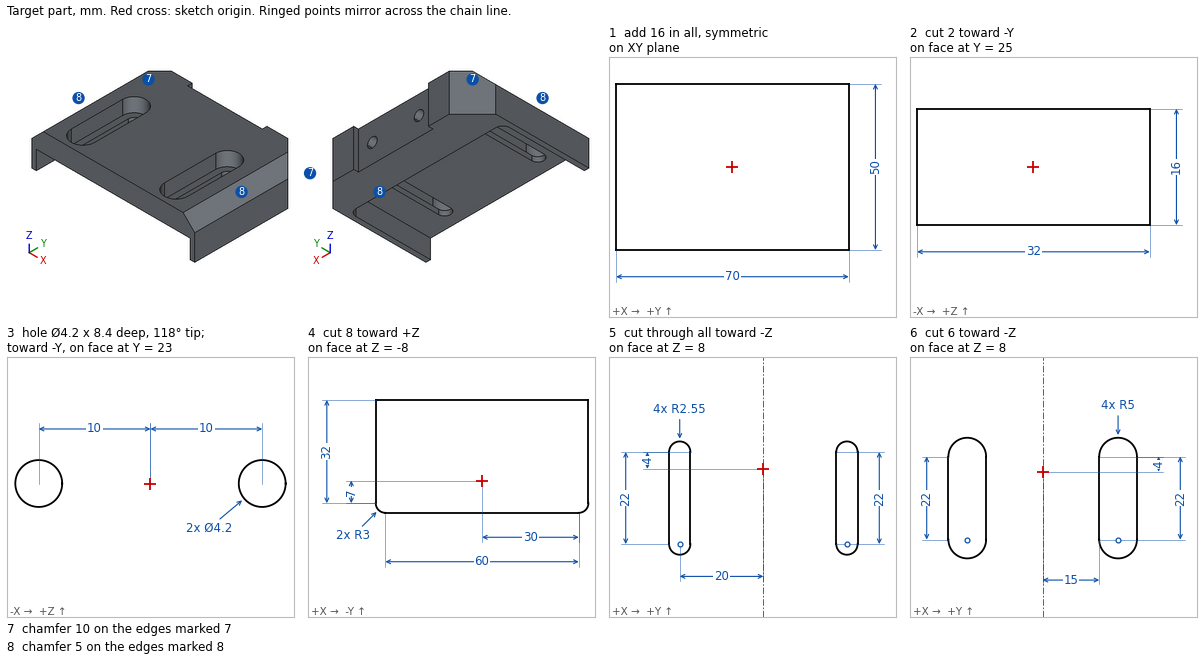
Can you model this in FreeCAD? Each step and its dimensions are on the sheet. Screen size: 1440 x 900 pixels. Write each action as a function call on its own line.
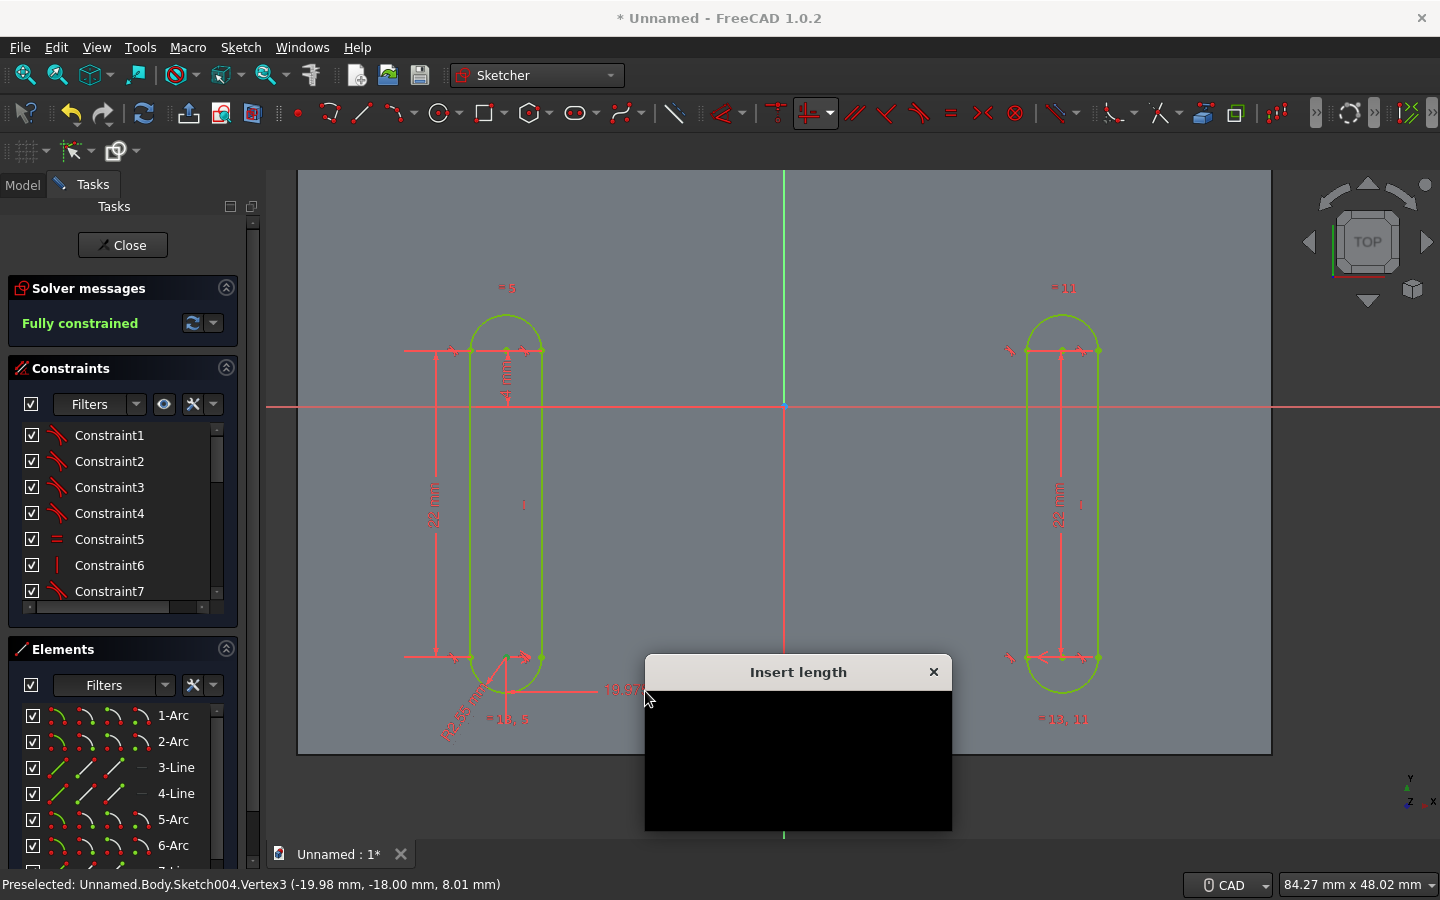
text(20)
key(Return)
key(Escape)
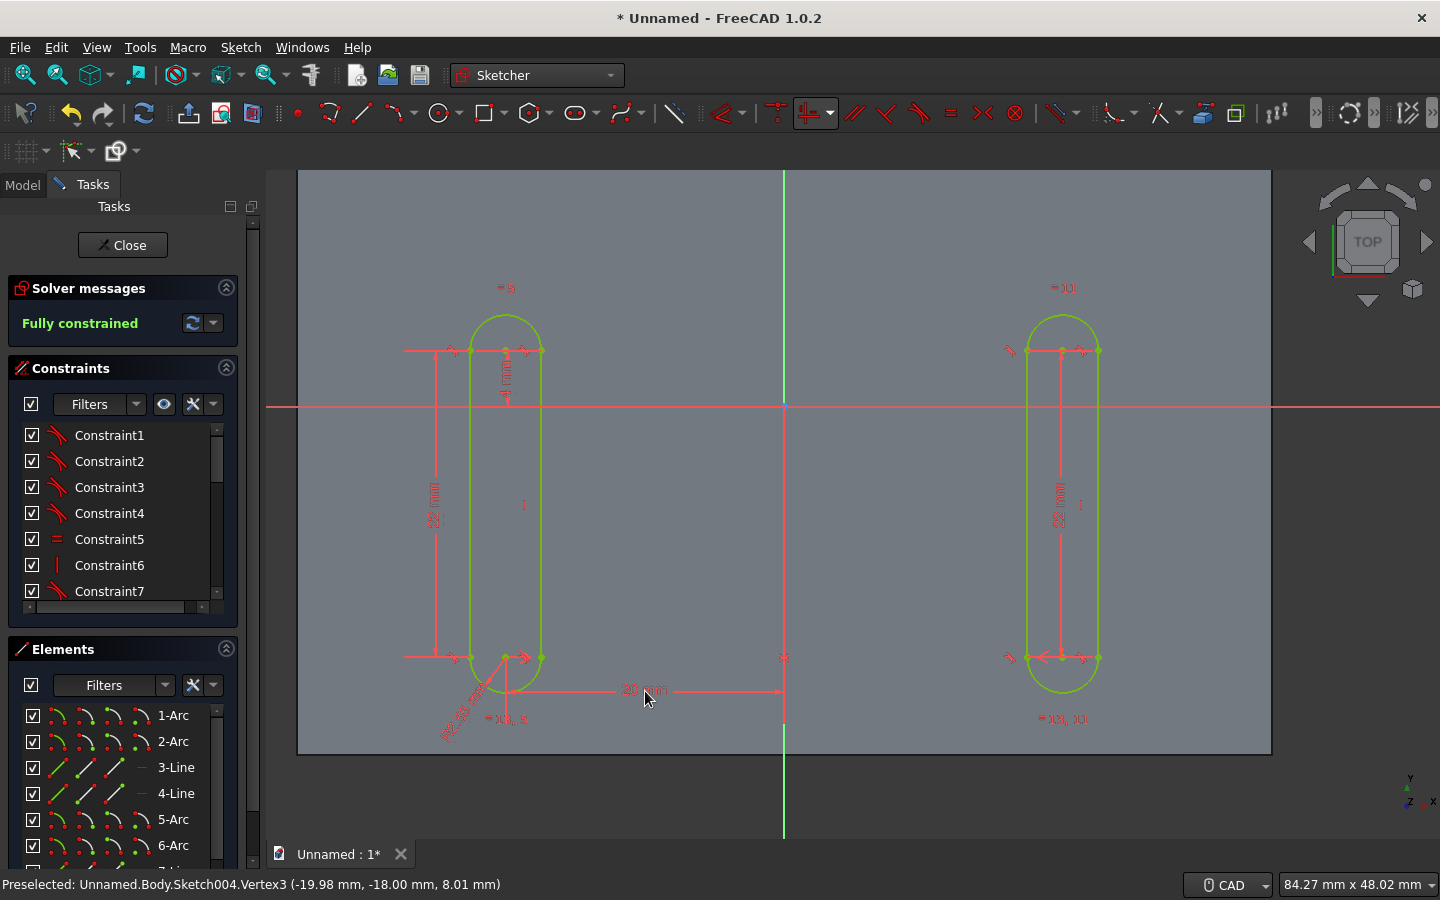
click(123, 245)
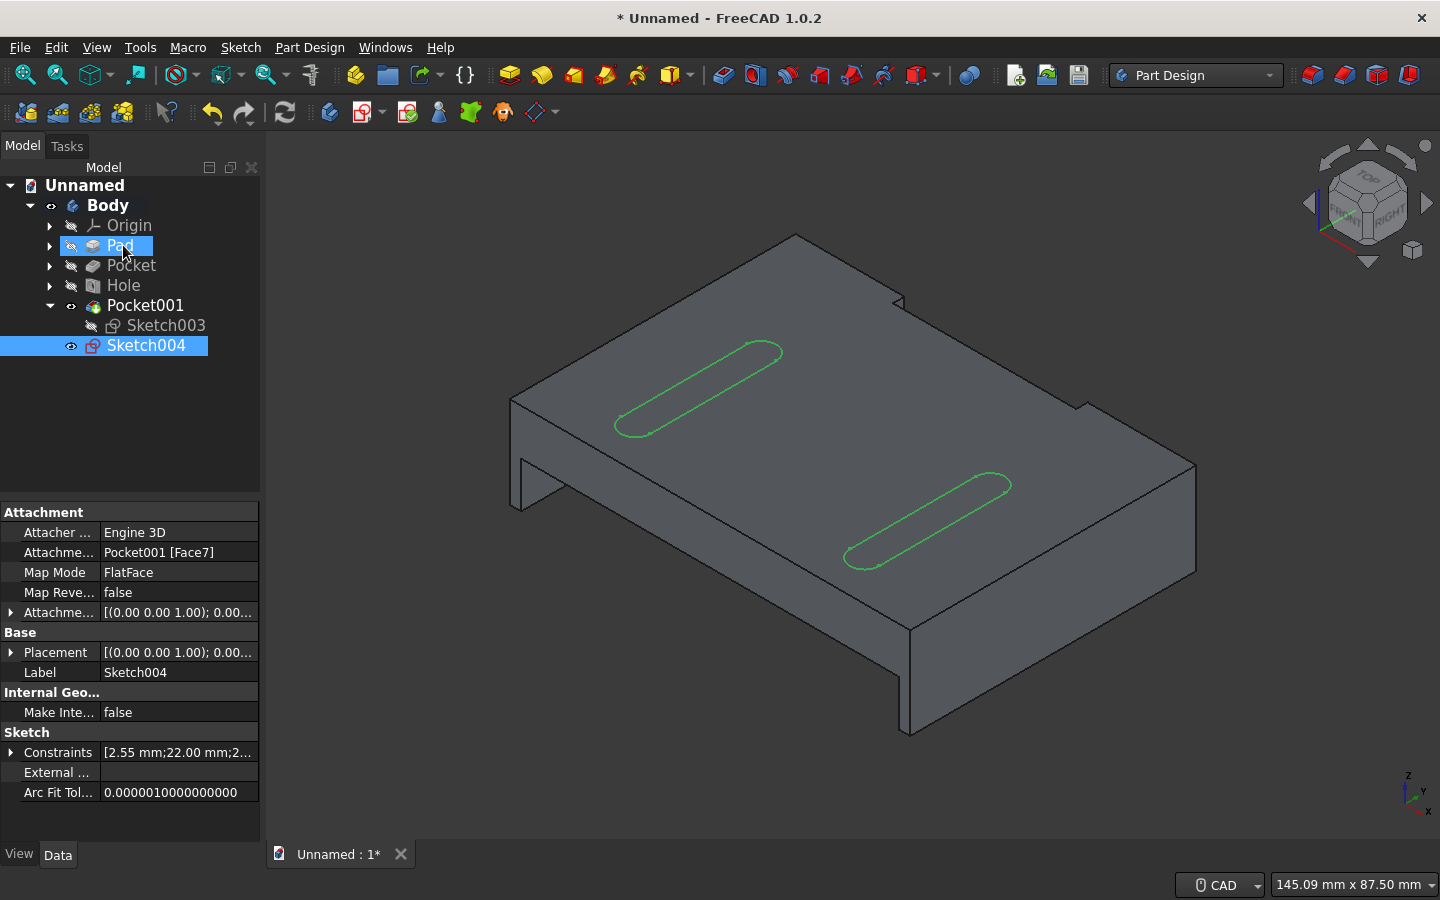
click(724, 76)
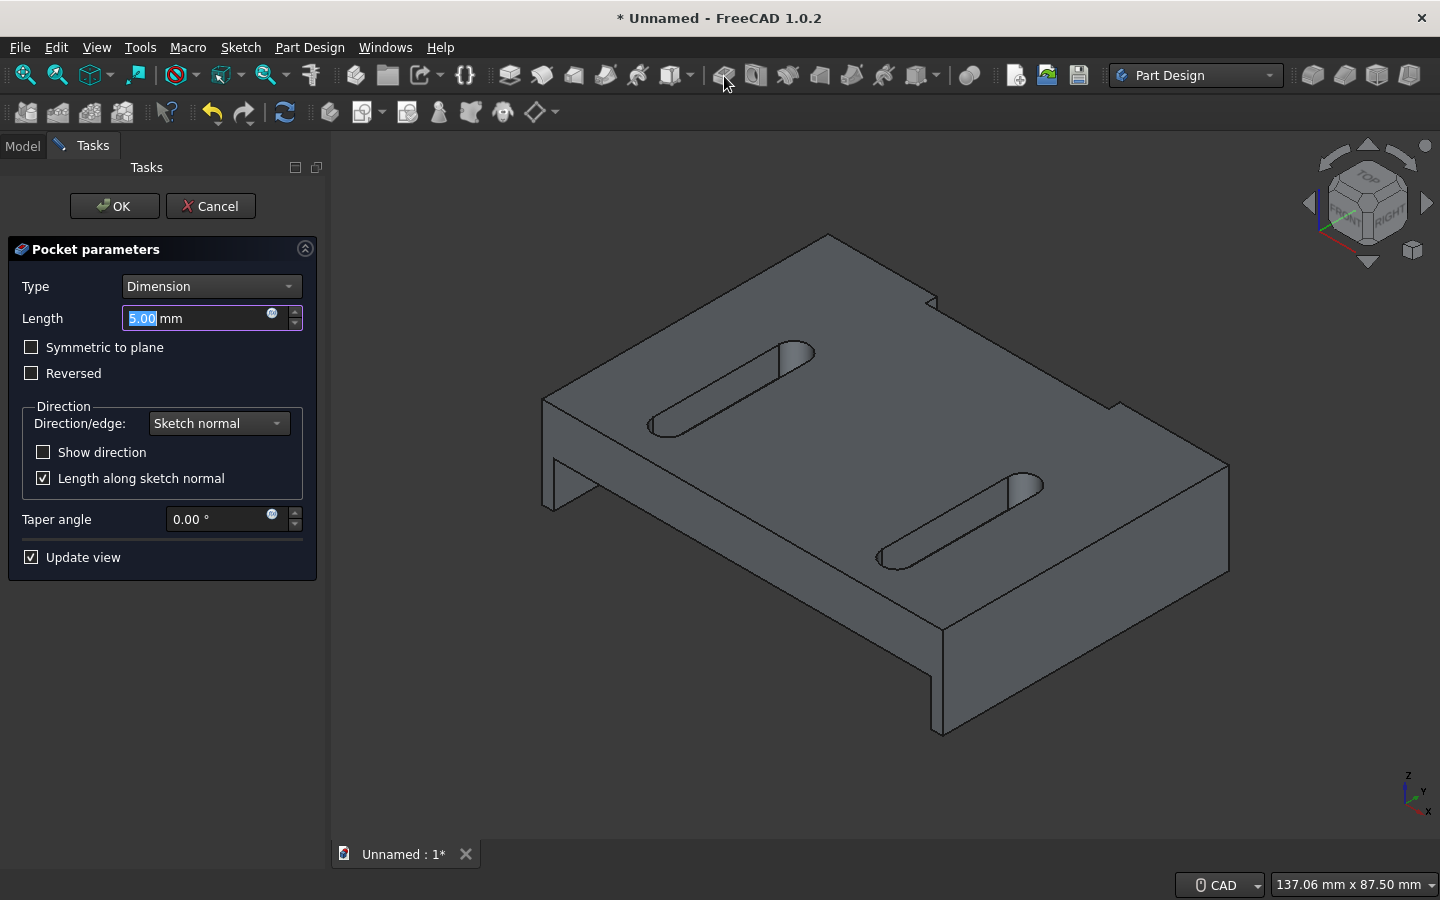
click(212, 286)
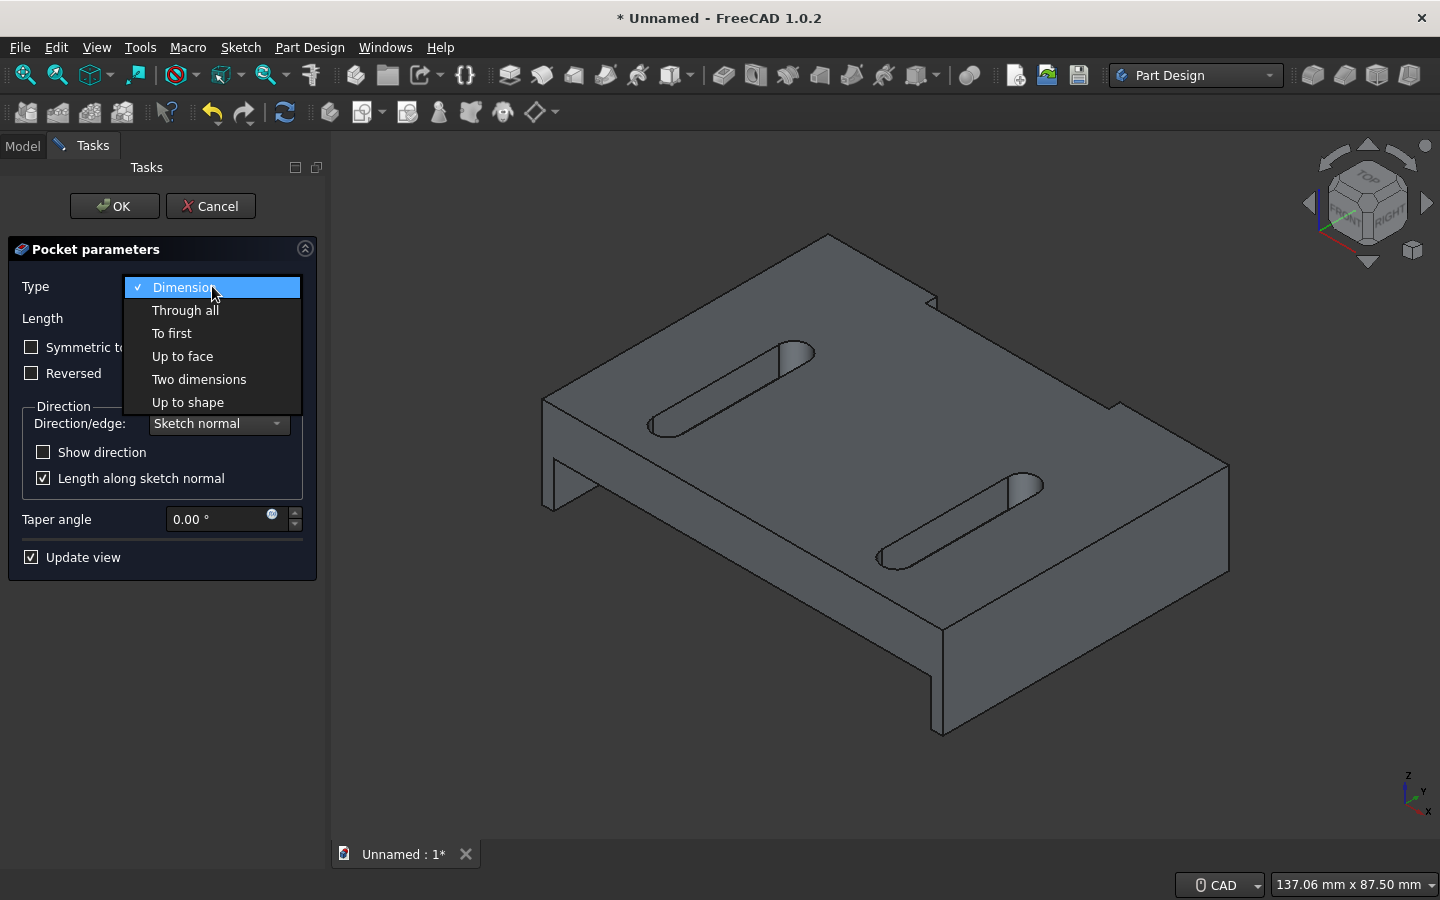
click(212, 310)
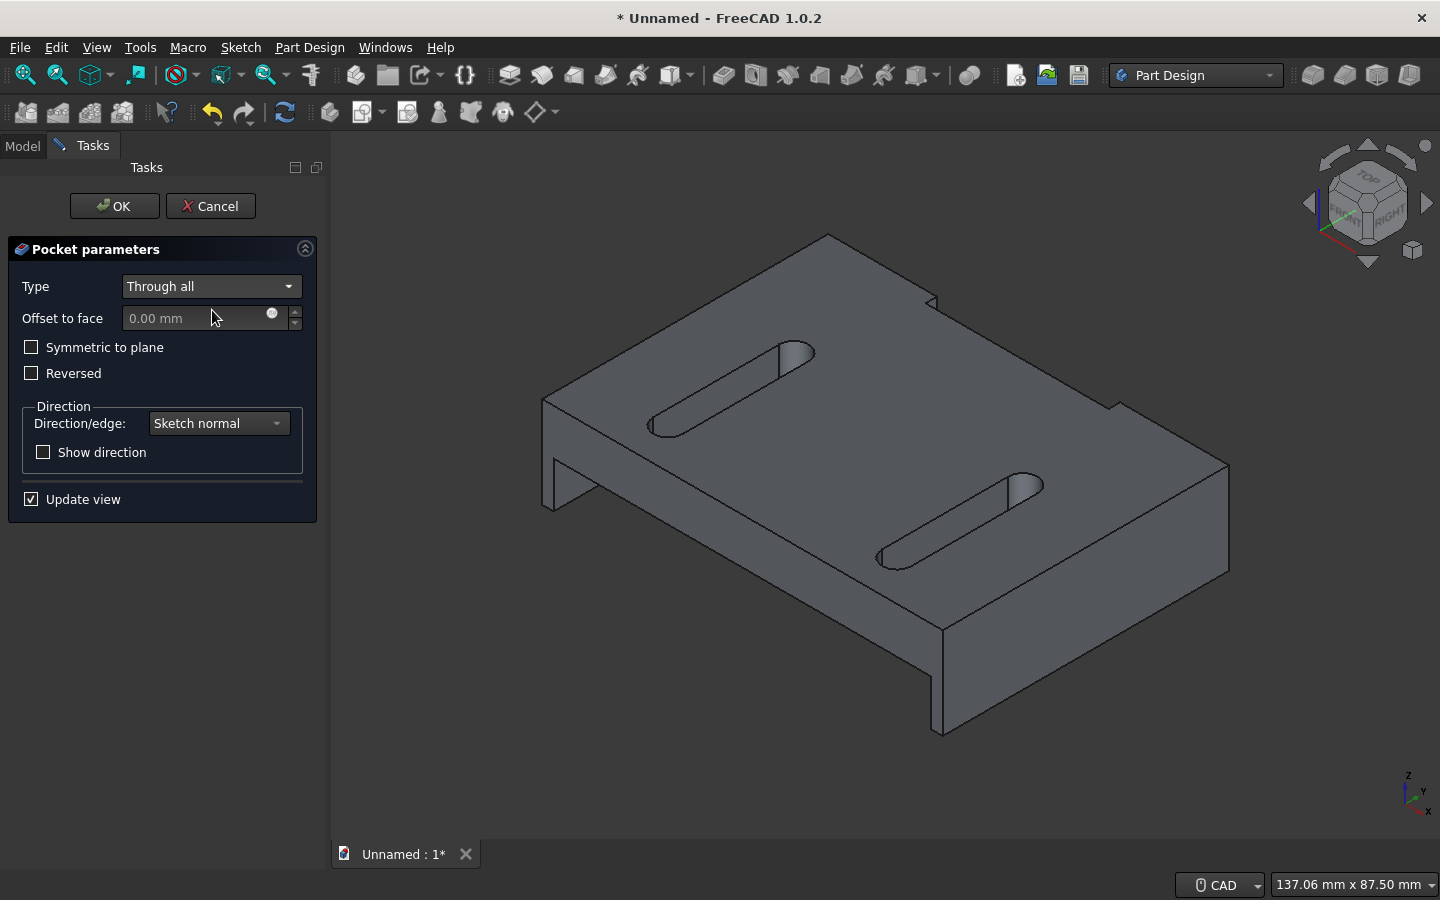
click(115, 206)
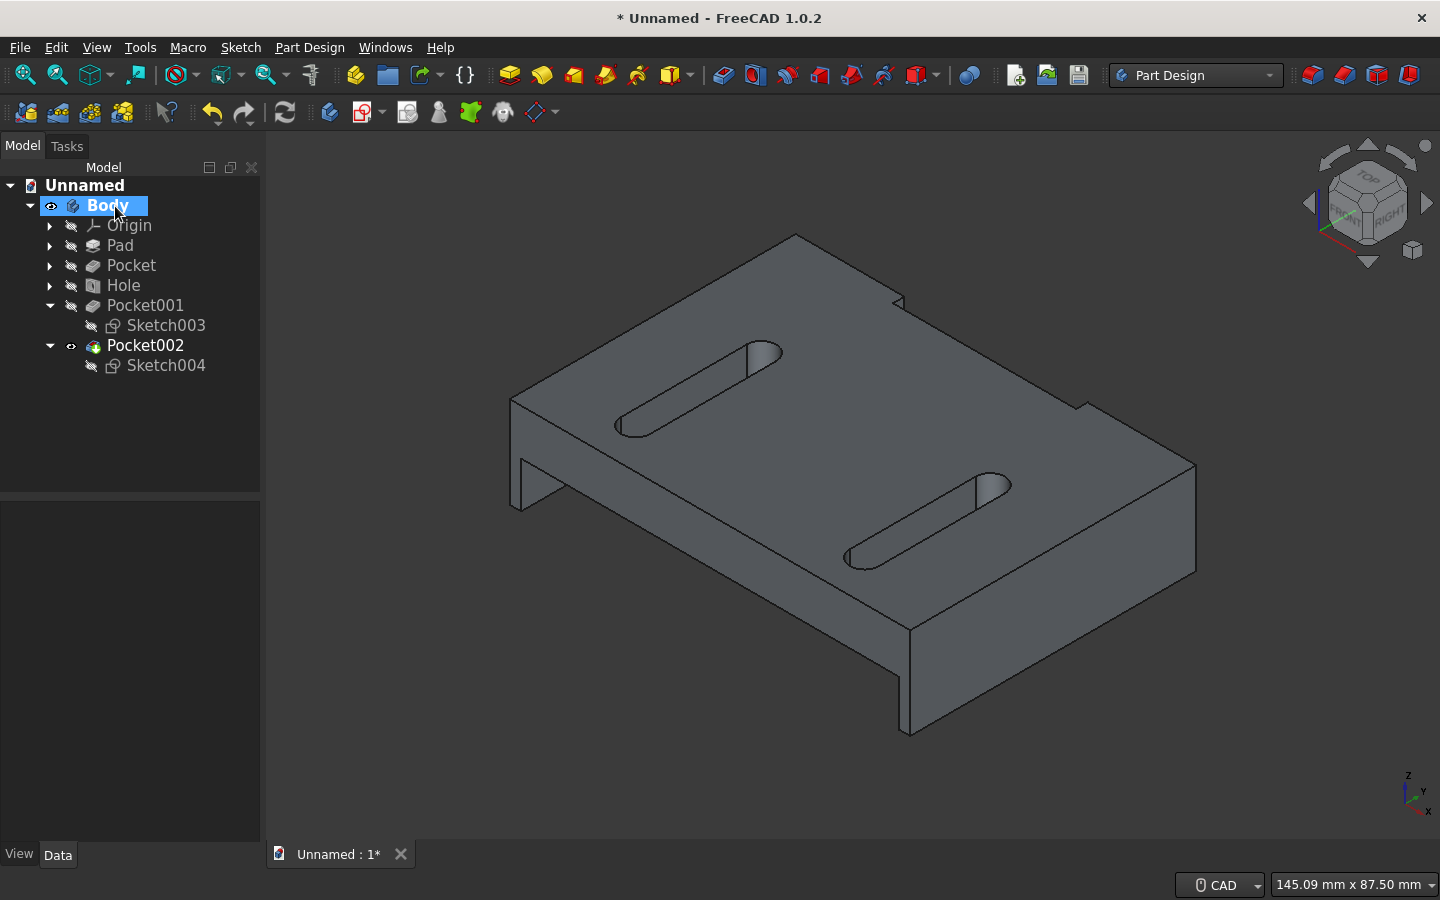
click(853, 431)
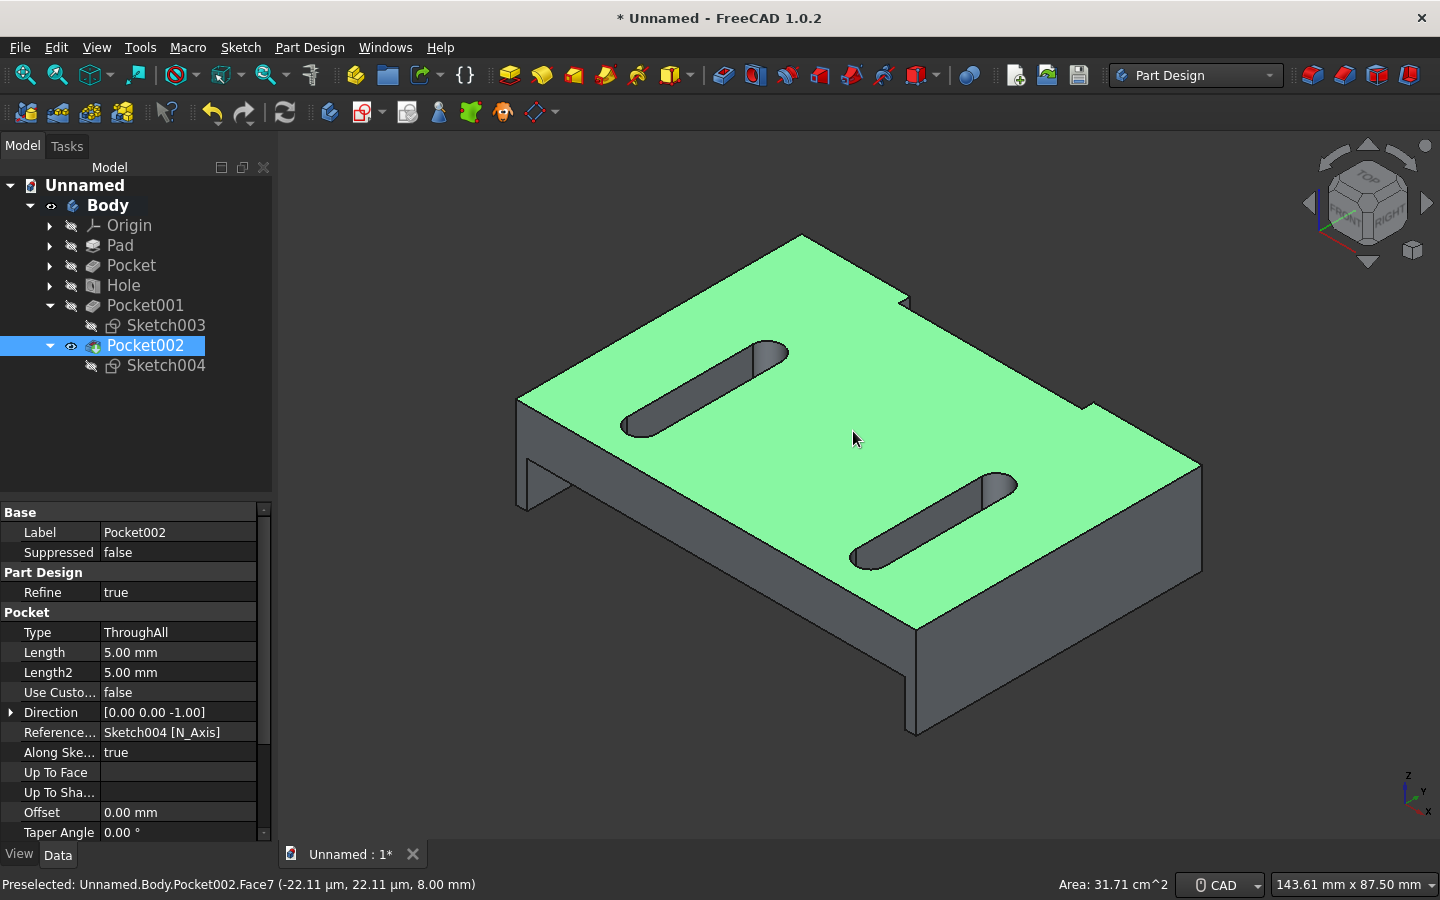
click(362, 112)